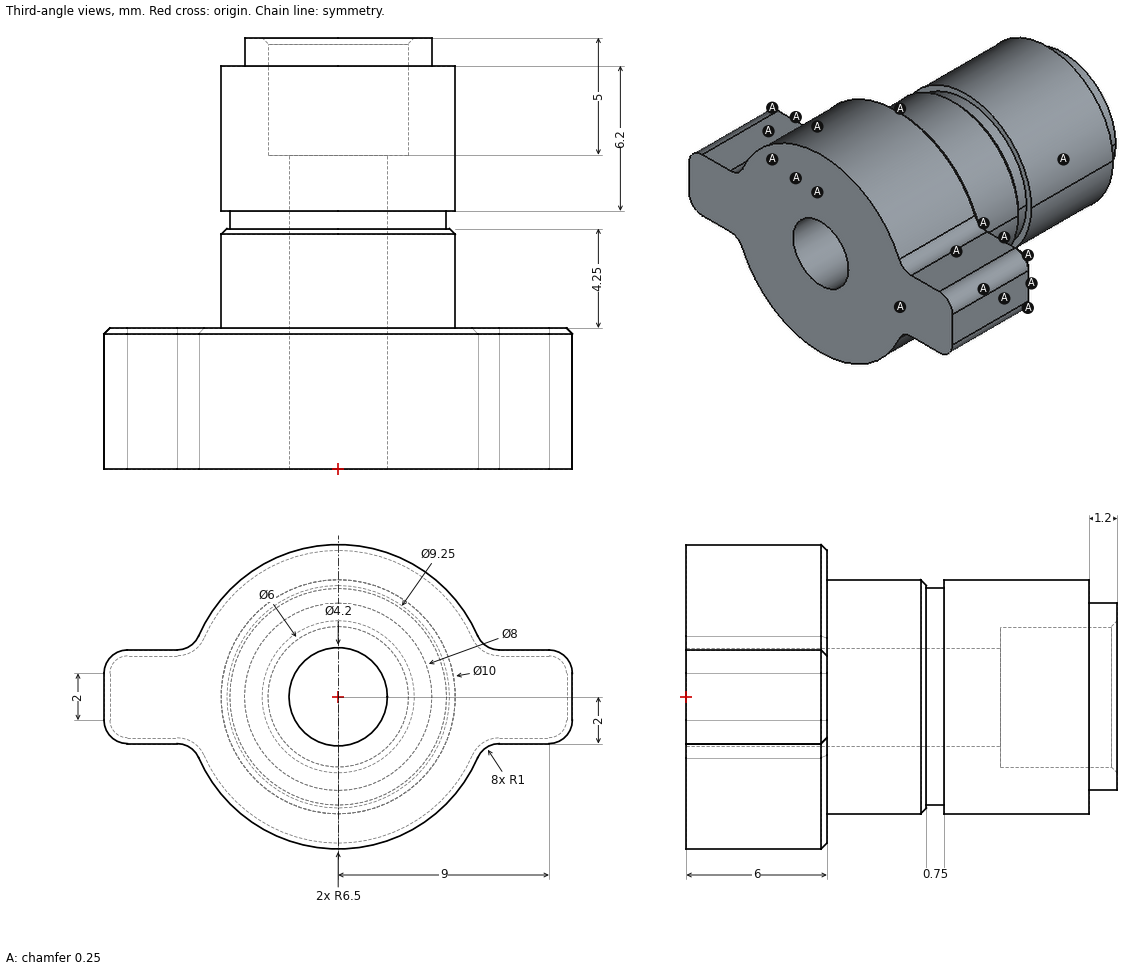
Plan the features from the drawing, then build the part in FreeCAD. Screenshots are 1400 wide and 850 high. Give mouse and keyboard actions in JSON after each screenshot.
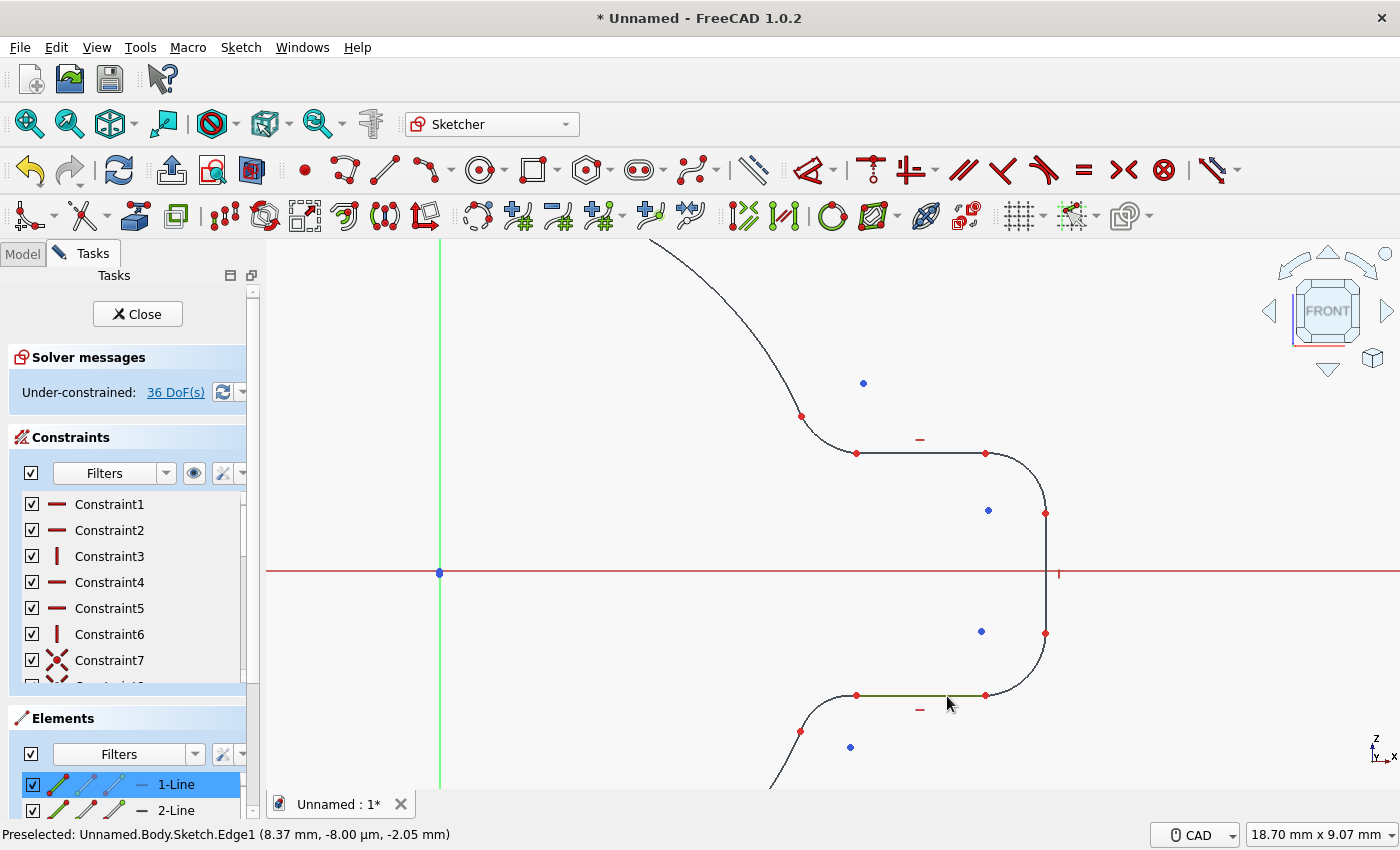
{"action": "left_click", "coordinate": [835, 698]}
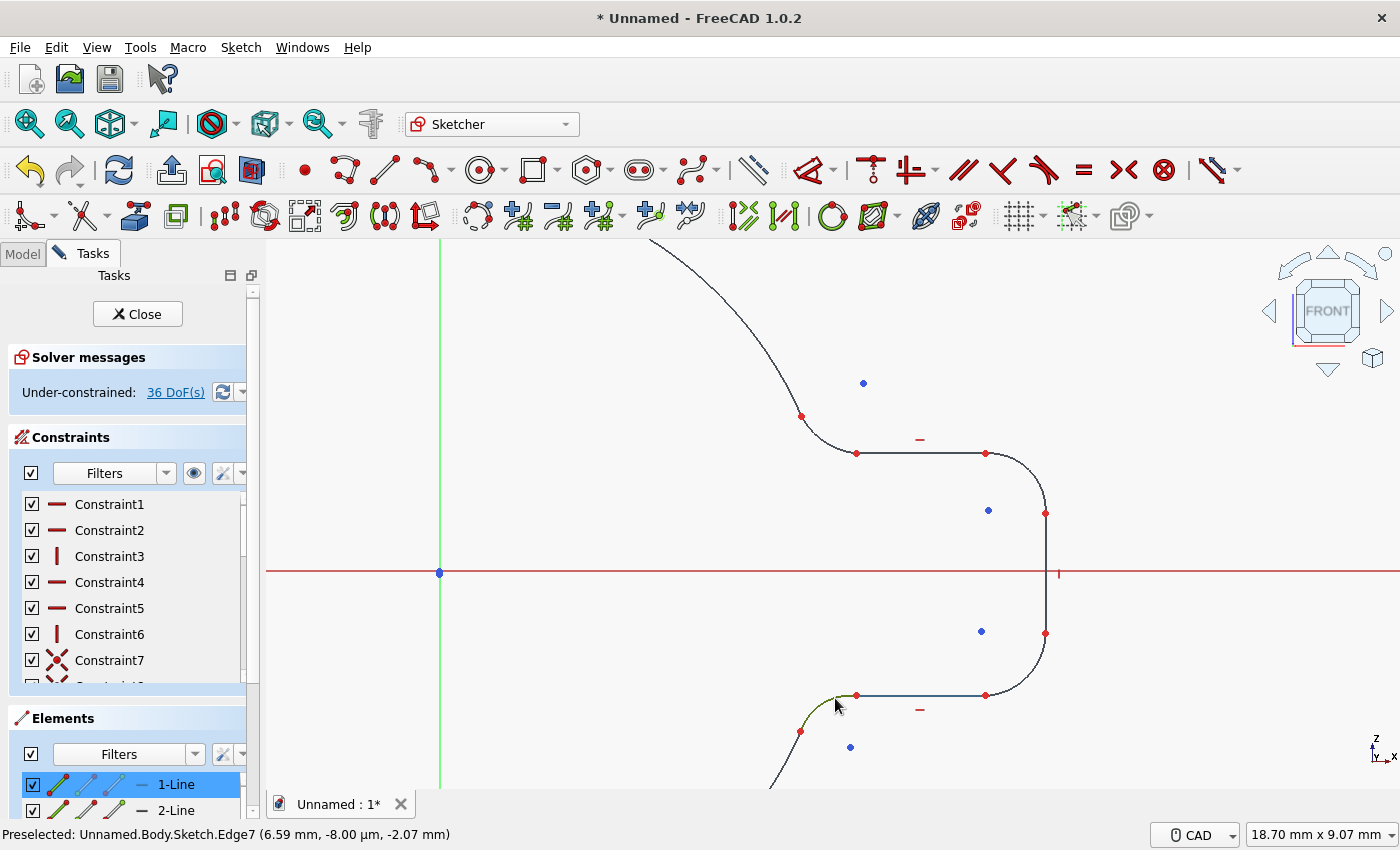
{"action": "left_click", "coordinate": [1044, 170]}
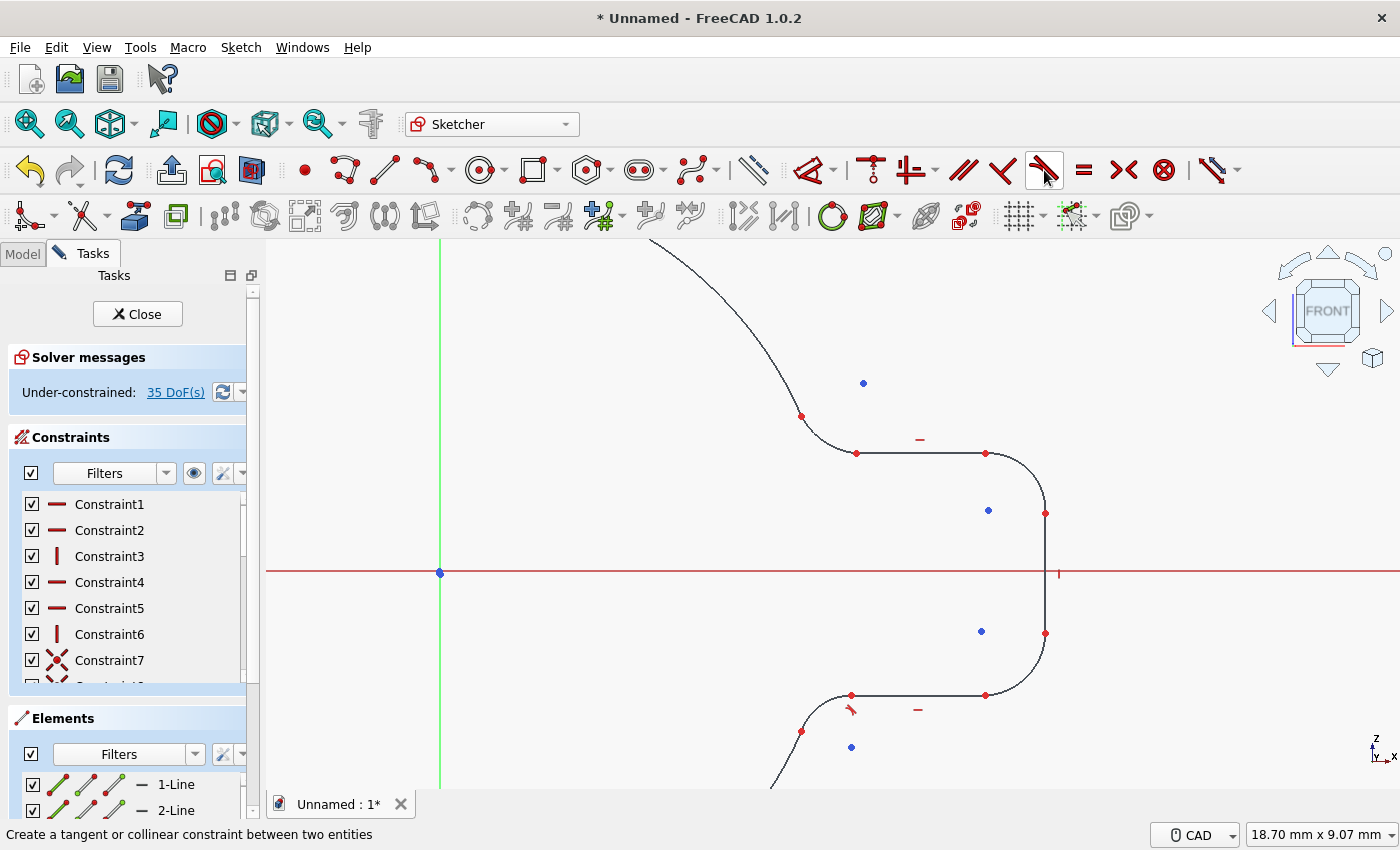
{"action": "left_click", "coordinate": [945, 696]}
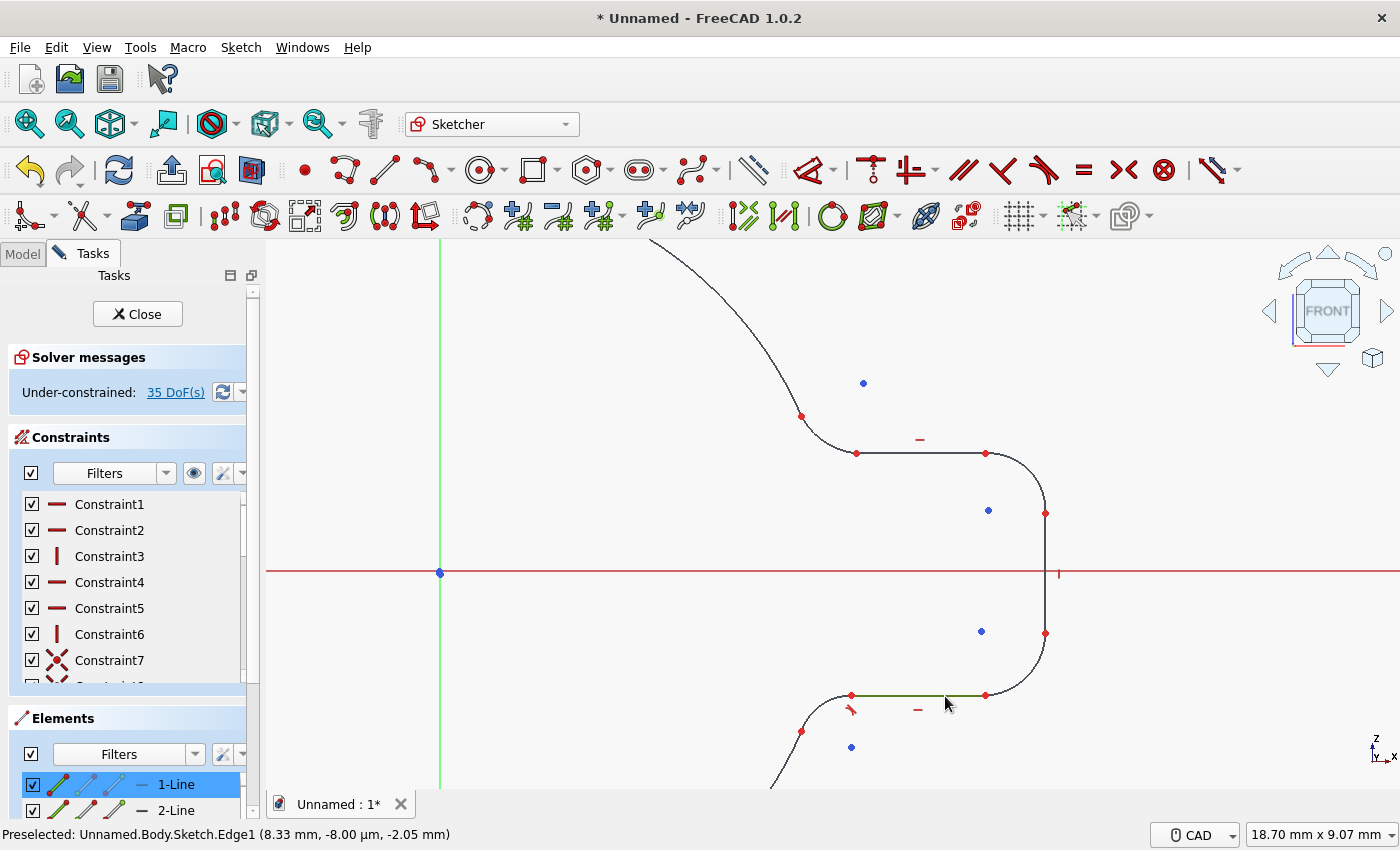
{"action": "left_click", "coordinate": [1012, 688]}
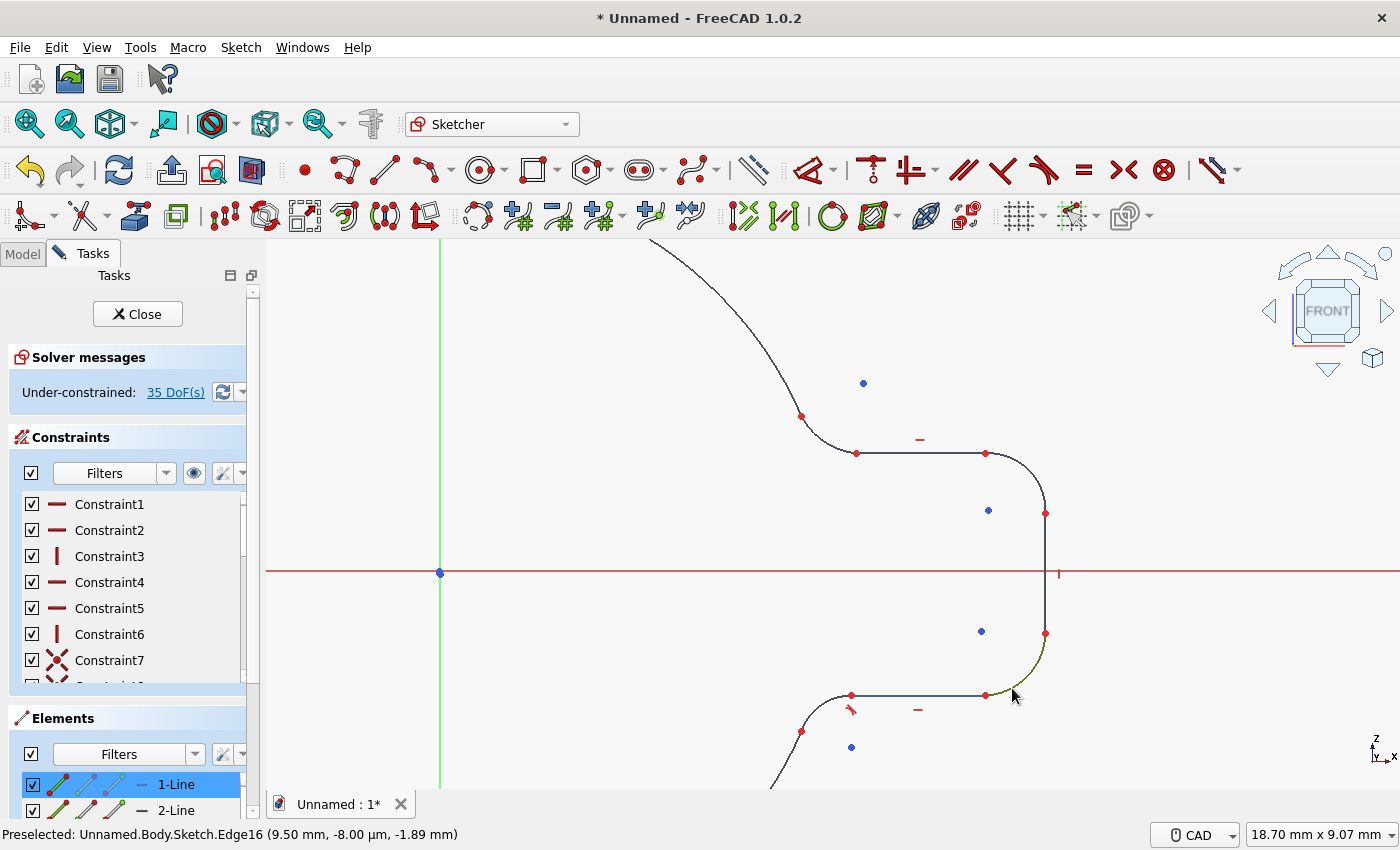
{"action": "left_click", "coordinate": [1044, 170]}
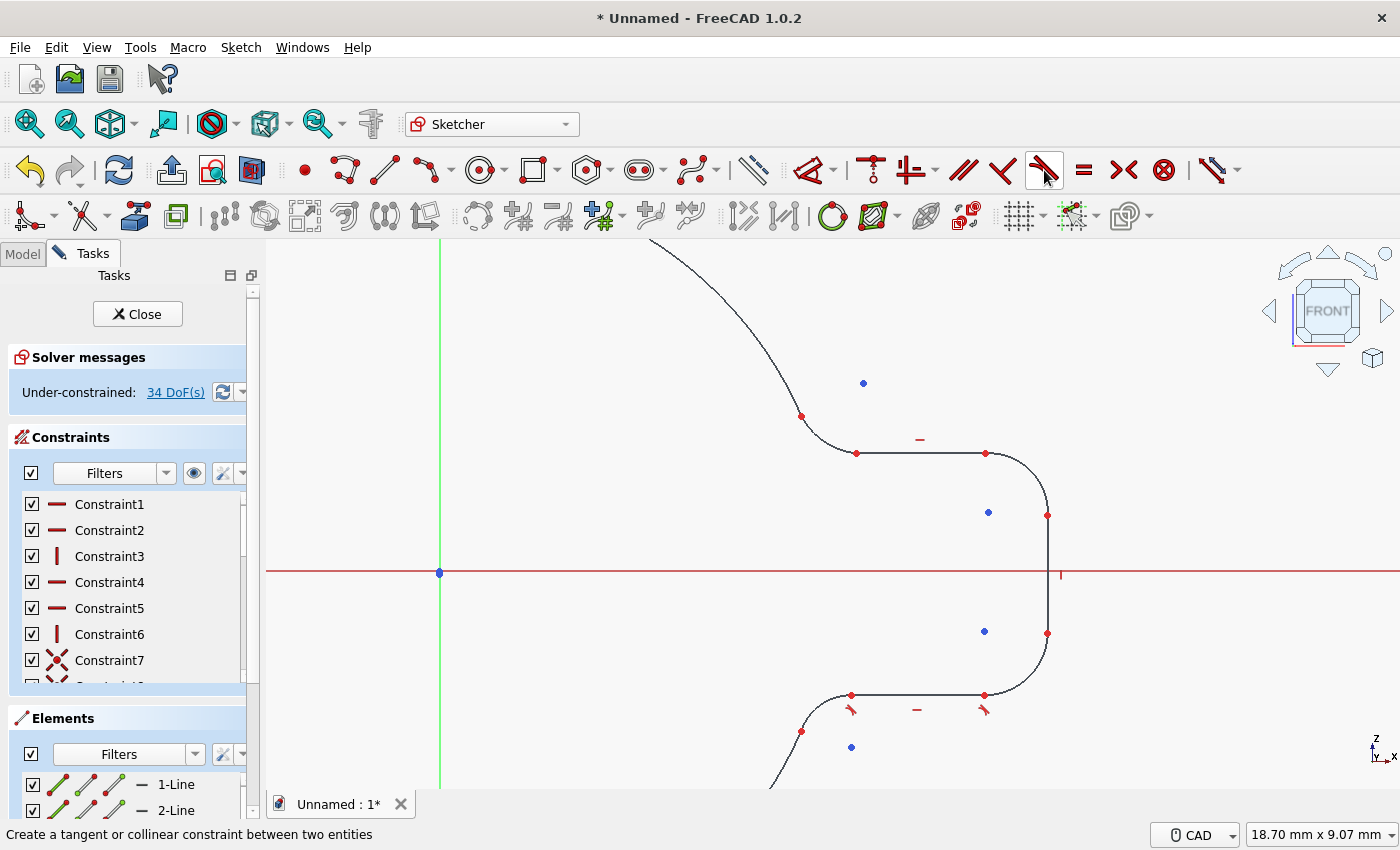
{"action": "scroll", "coordinate": [1030, 467], "scroll_direction": "down", "scroll_amount": 4}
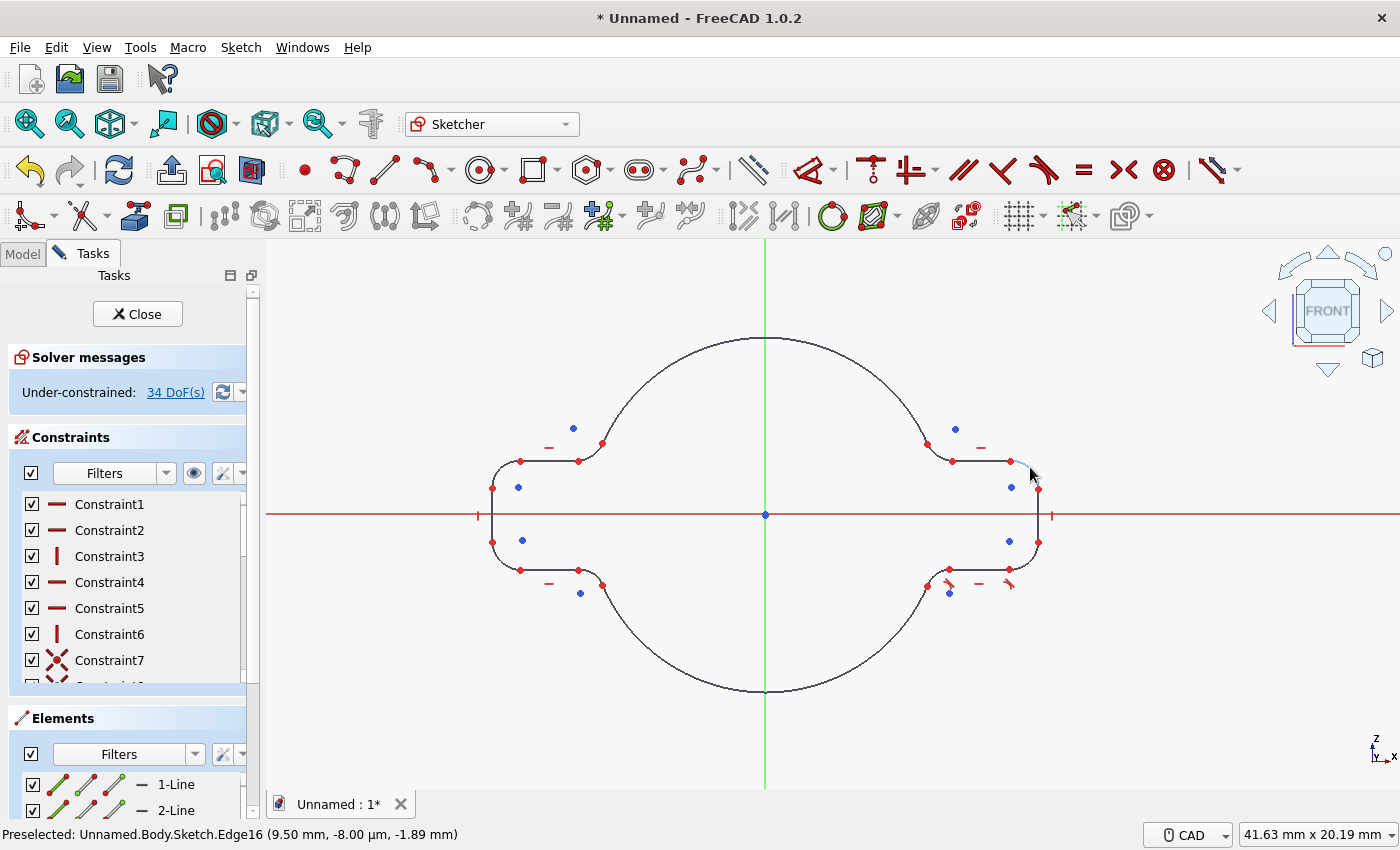
{"action": "left_click", "coordinate": [561, 570]}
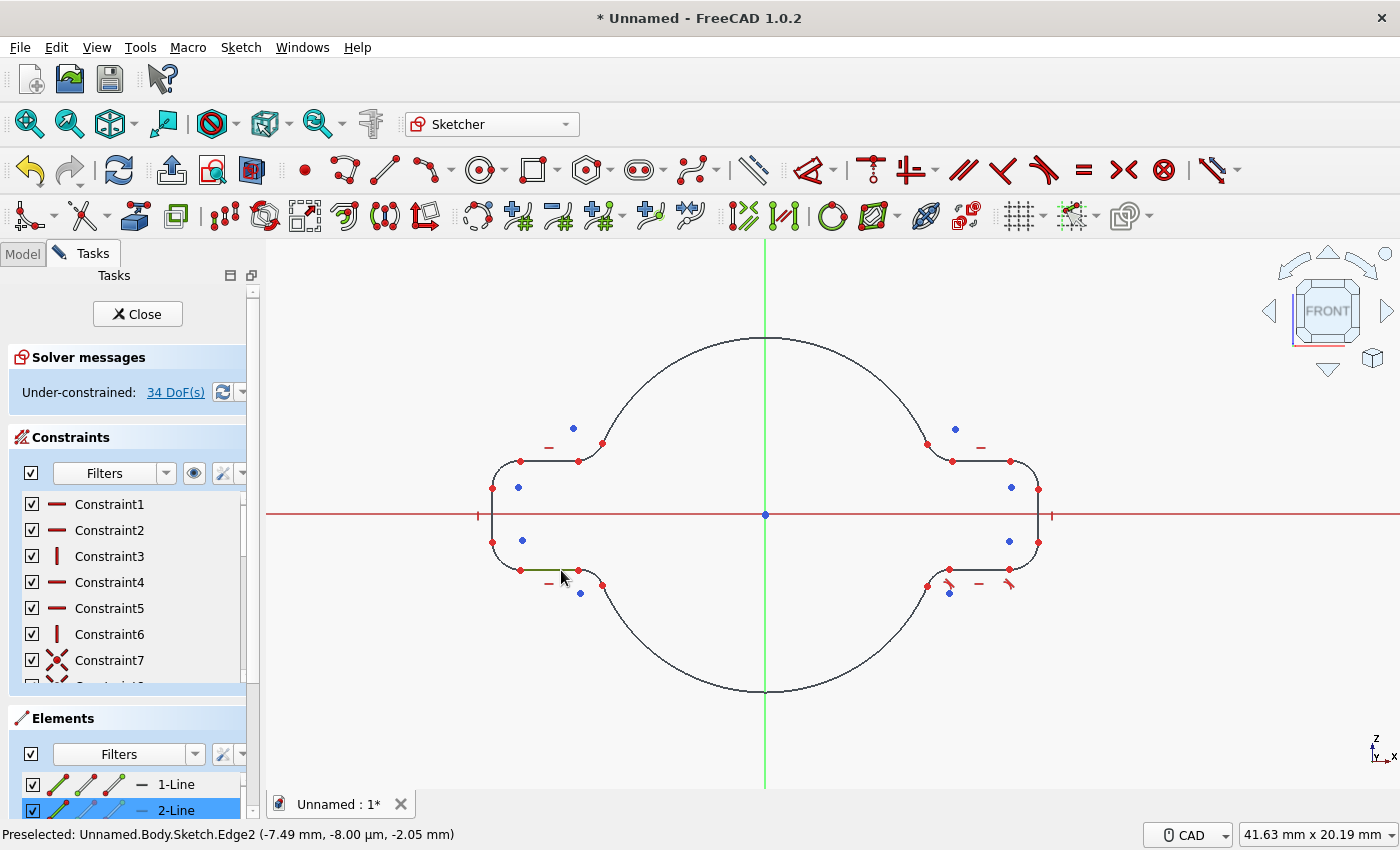
{"action": "scroll", "coordinate": [598, 578], "scroll_direction": "up", "scroll_amount": 2}